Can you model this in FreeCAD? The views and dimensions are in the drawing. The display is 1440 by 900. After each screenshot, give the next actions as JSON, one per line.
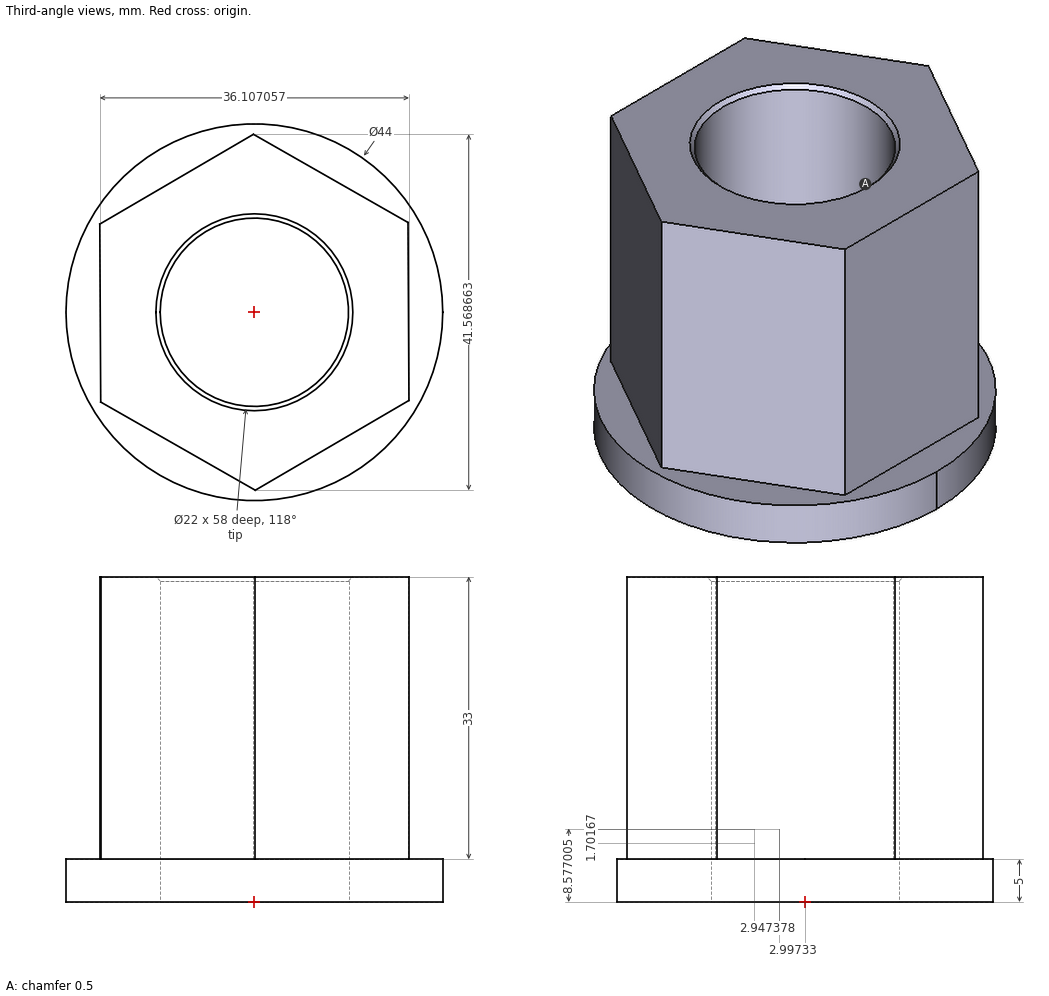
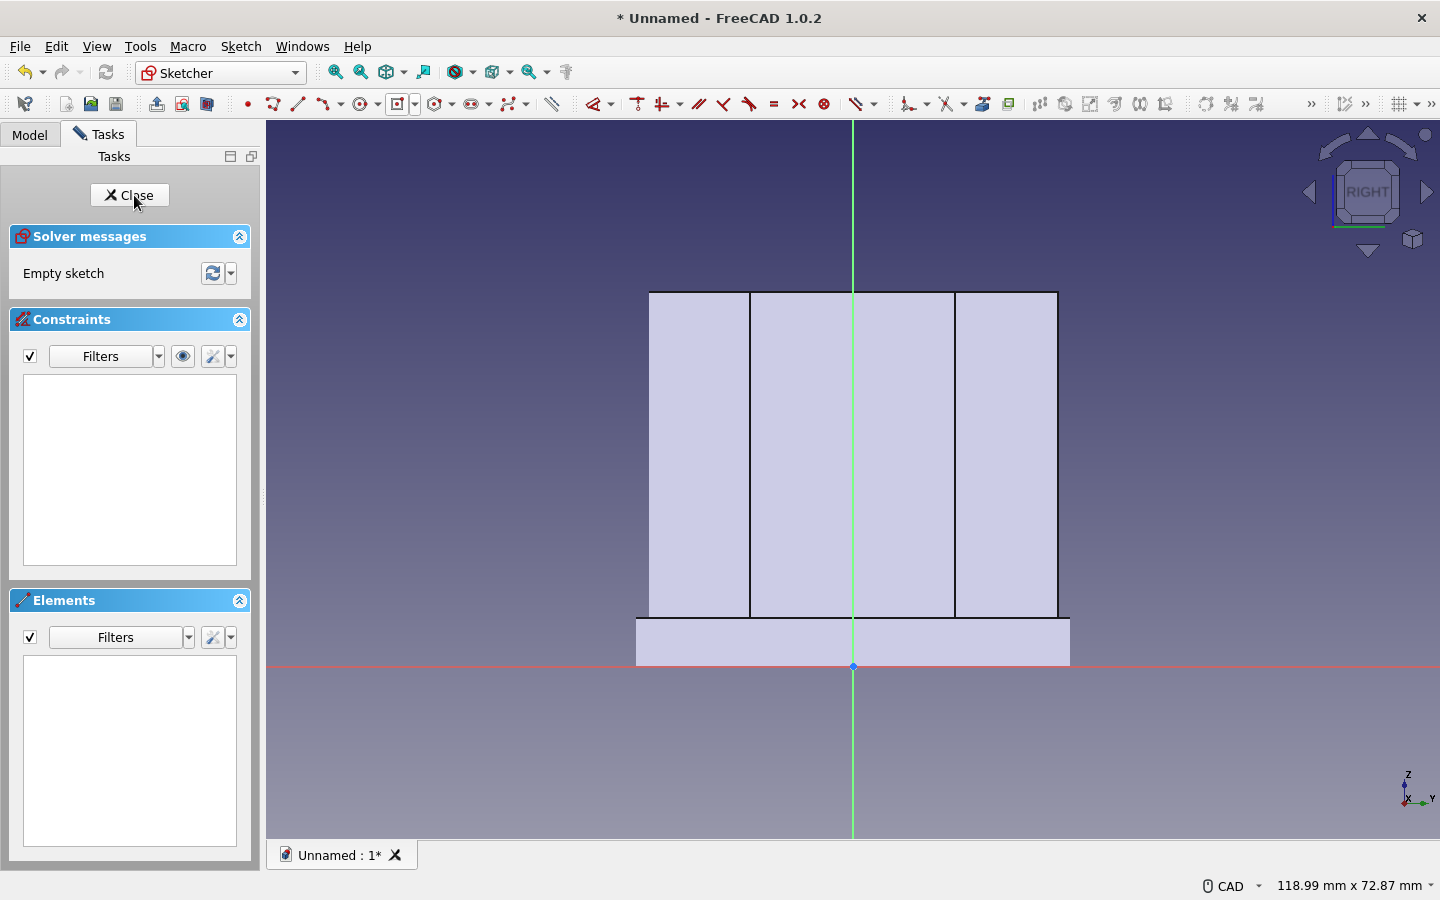
{"action": "scroll", "coordinate": [810, 597], "scroll_direction": "up", "scroll_amount": 15}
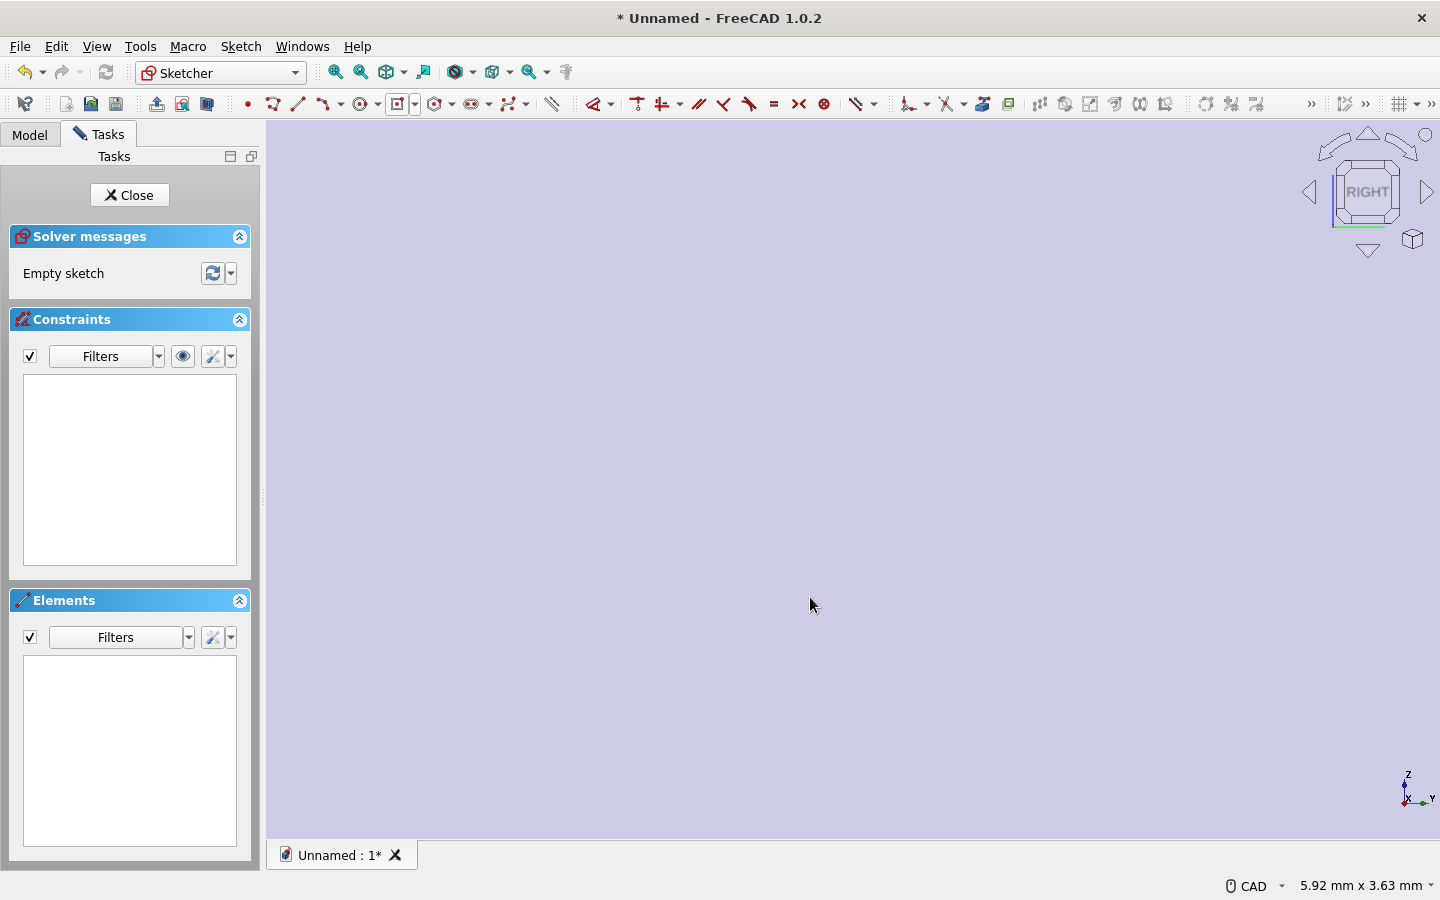
{"action": "left_click", "coordinate": [273, 104]}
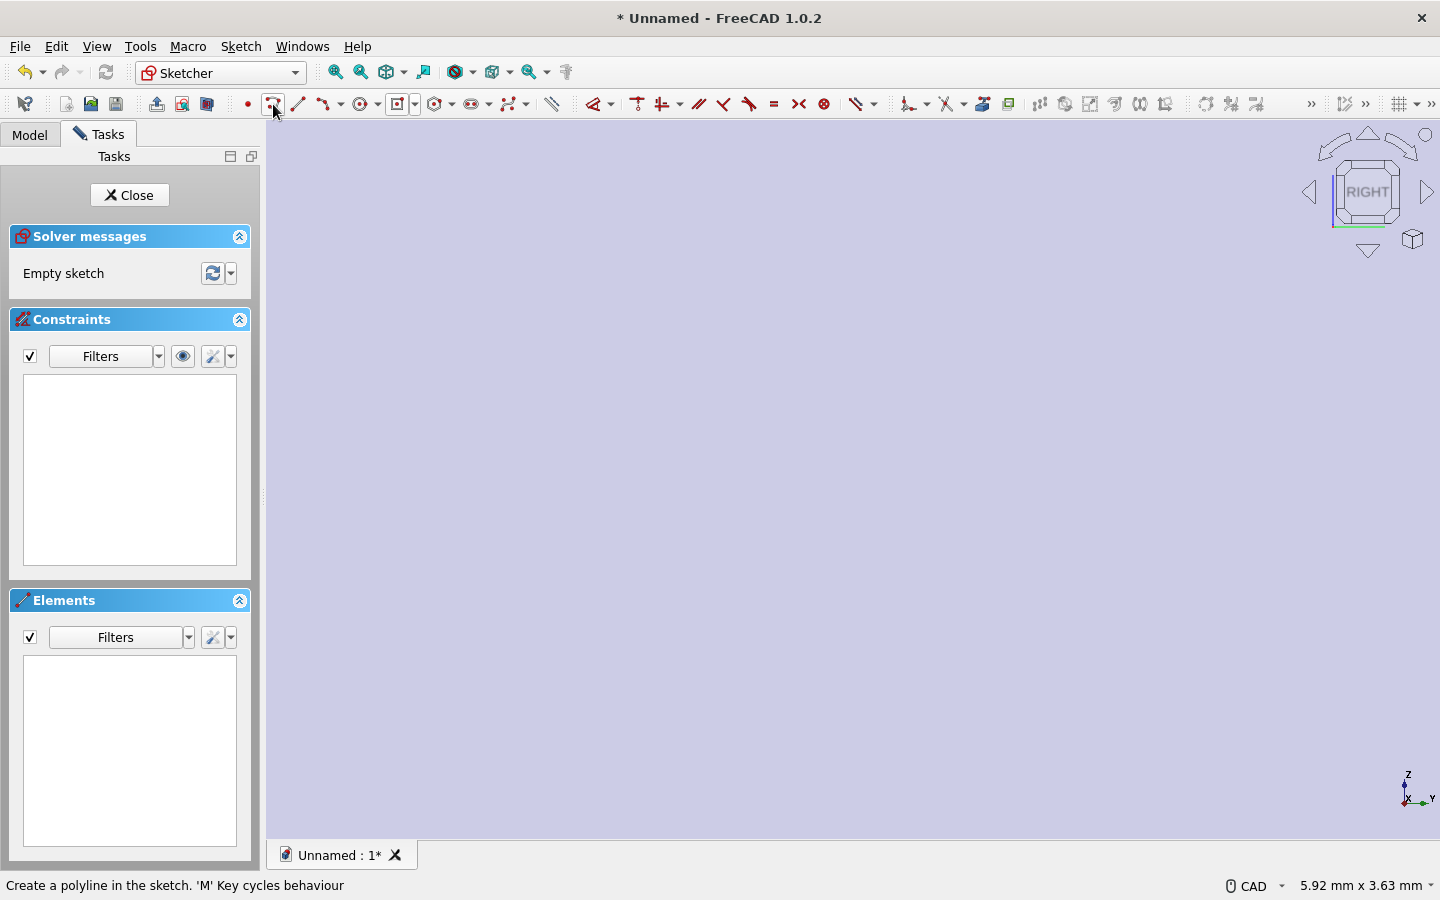
{"action": "left_click", "coordinate": [1071, 290]}
{"action": "left_click", "coordinate": [487, 290]}
{"action": "left_click", "coordinate": [487, 627]}
{"action": "left_click", "coordinate": [1071, 291]}
{"action": "key", "text": "Escape"}
{"action": "key", "text": "Escape"}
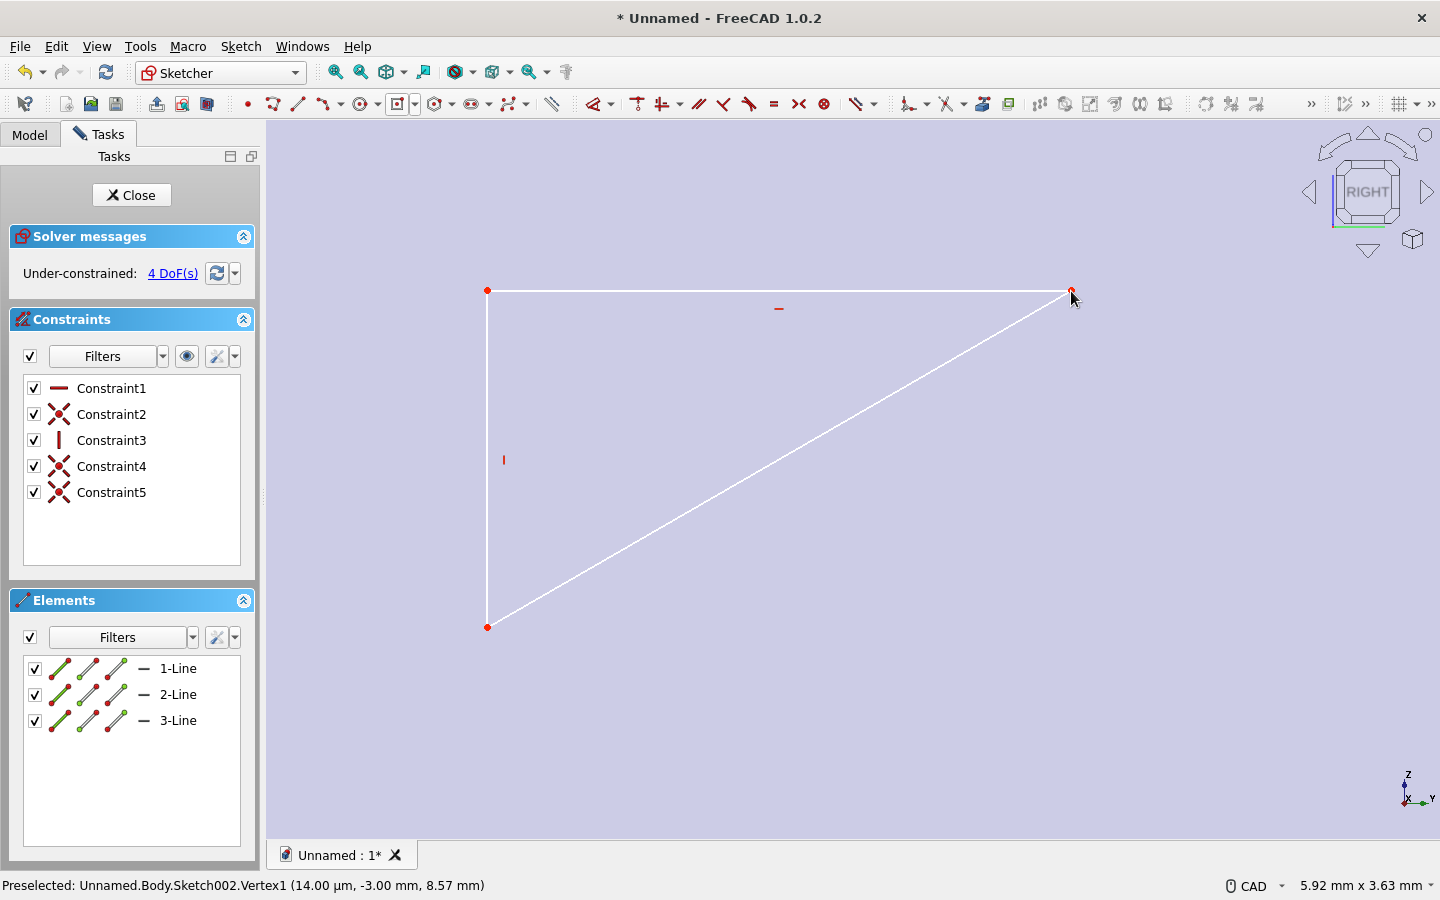
{"action": "left_click", "coordinate": [487, 392]}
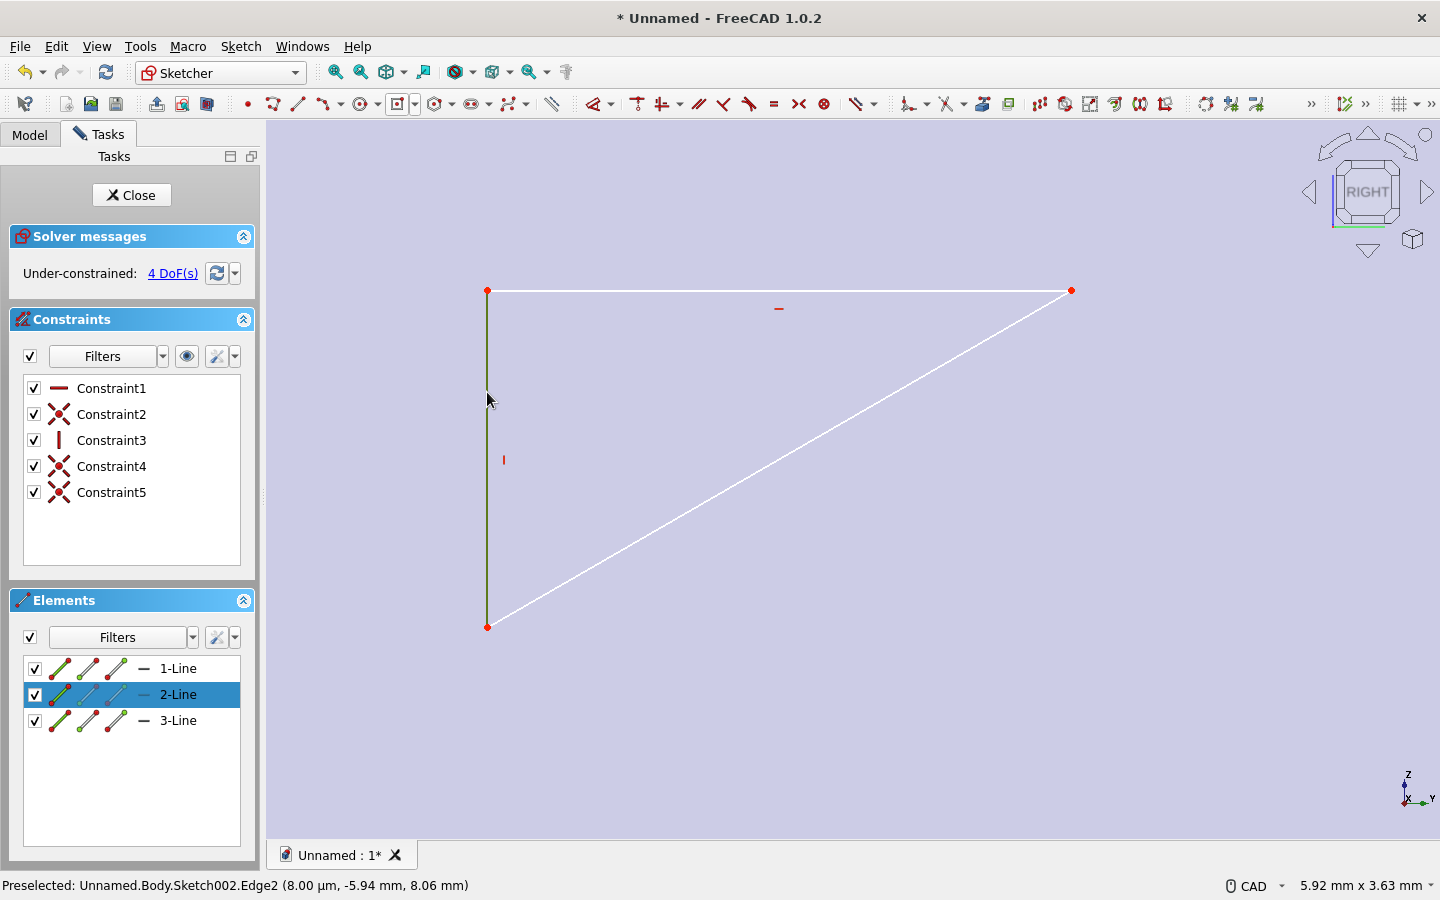
{"action": "key", "text": "i"}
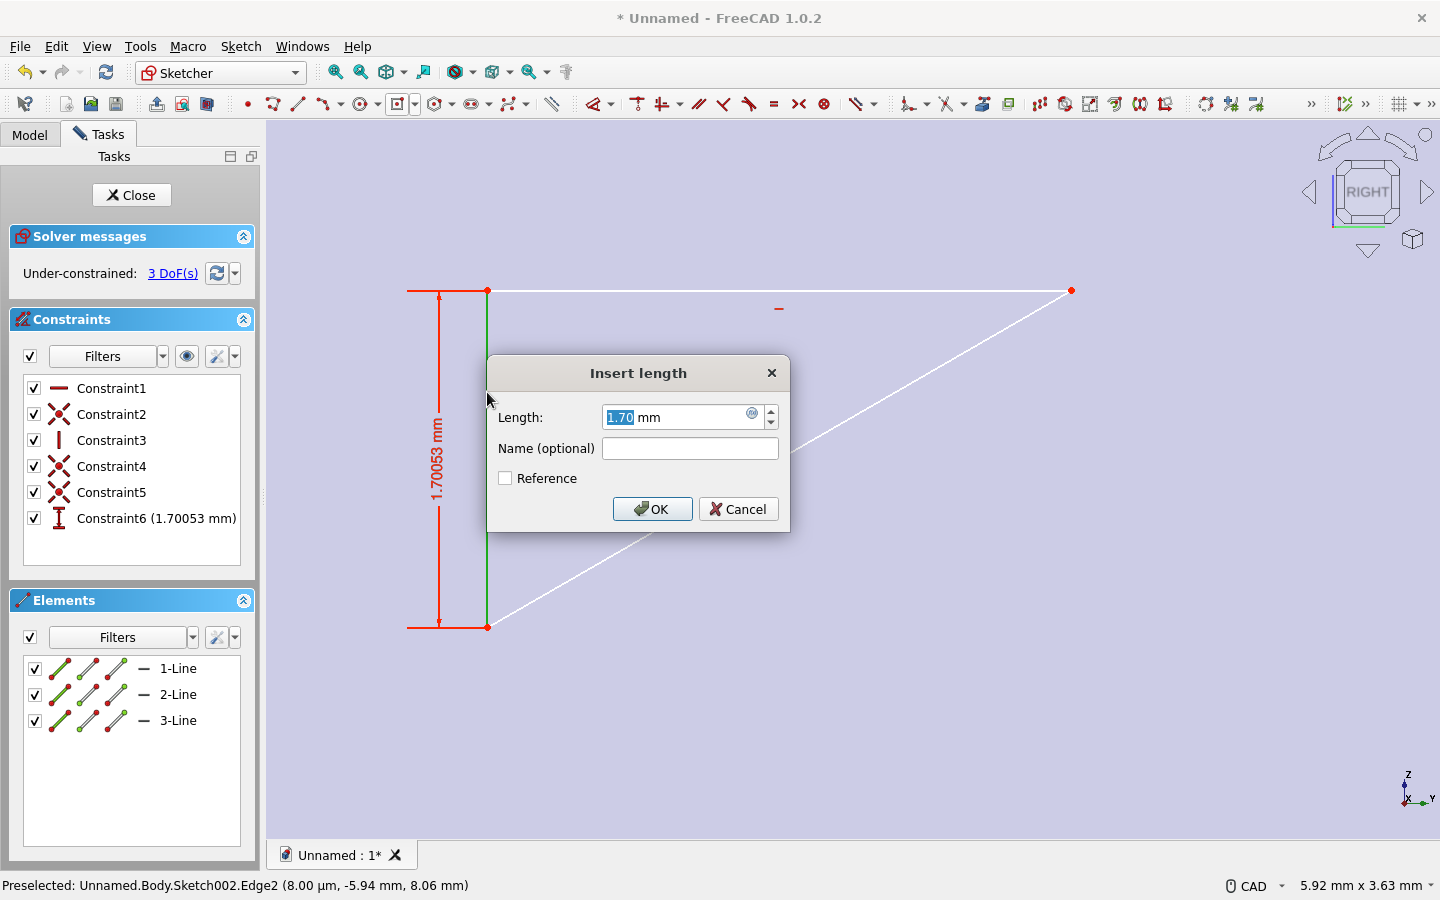
{"action": "type", "text": "1.70167"}
{"action": "key", "text": "Return"}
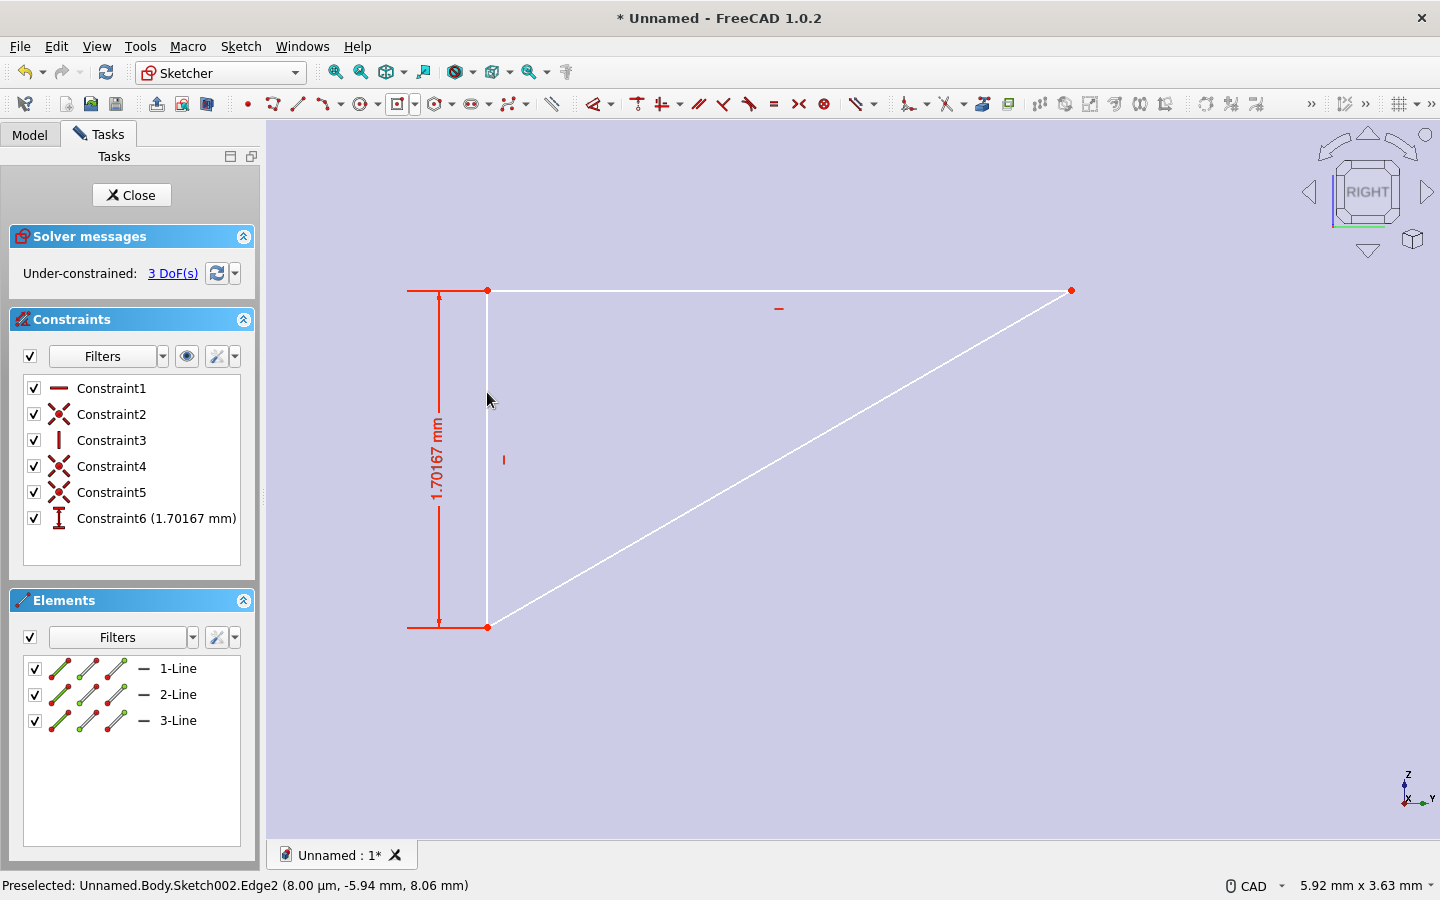
{"action": "left_click", "coordinate": [896, 291]}